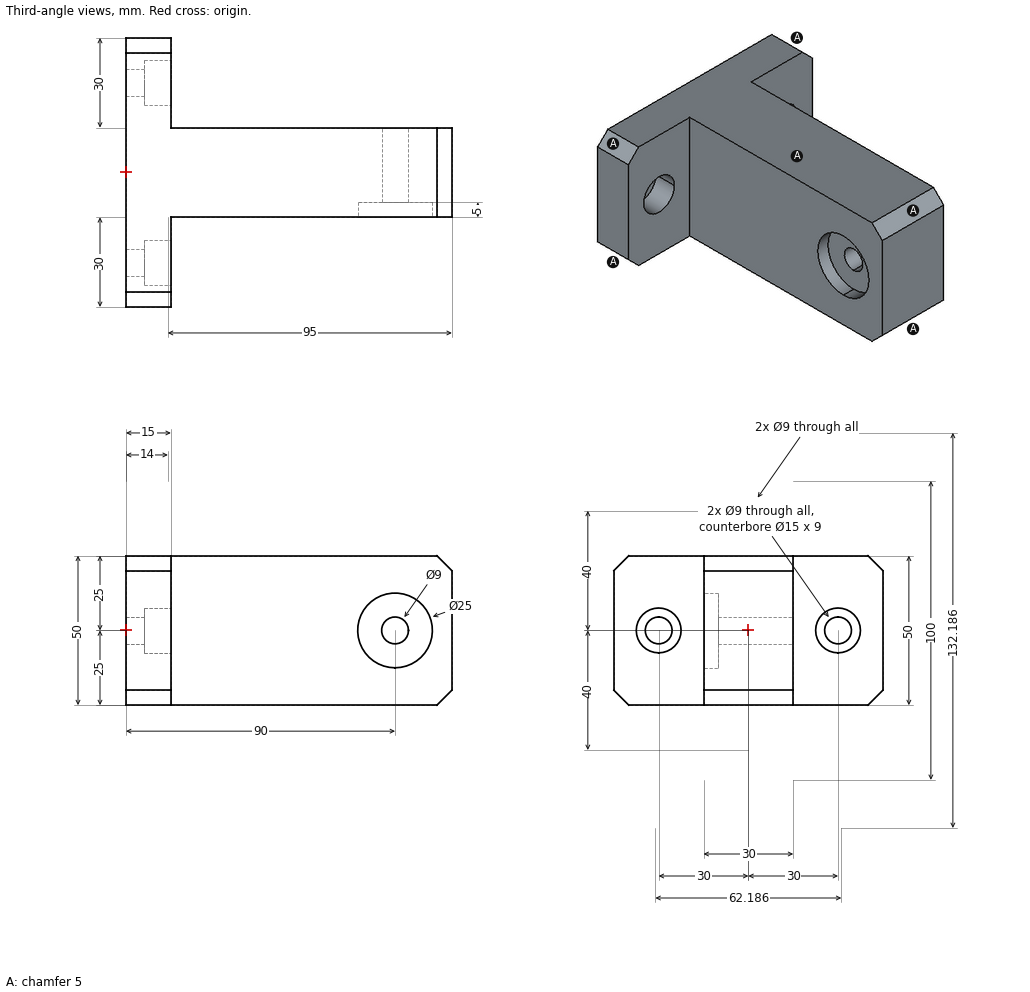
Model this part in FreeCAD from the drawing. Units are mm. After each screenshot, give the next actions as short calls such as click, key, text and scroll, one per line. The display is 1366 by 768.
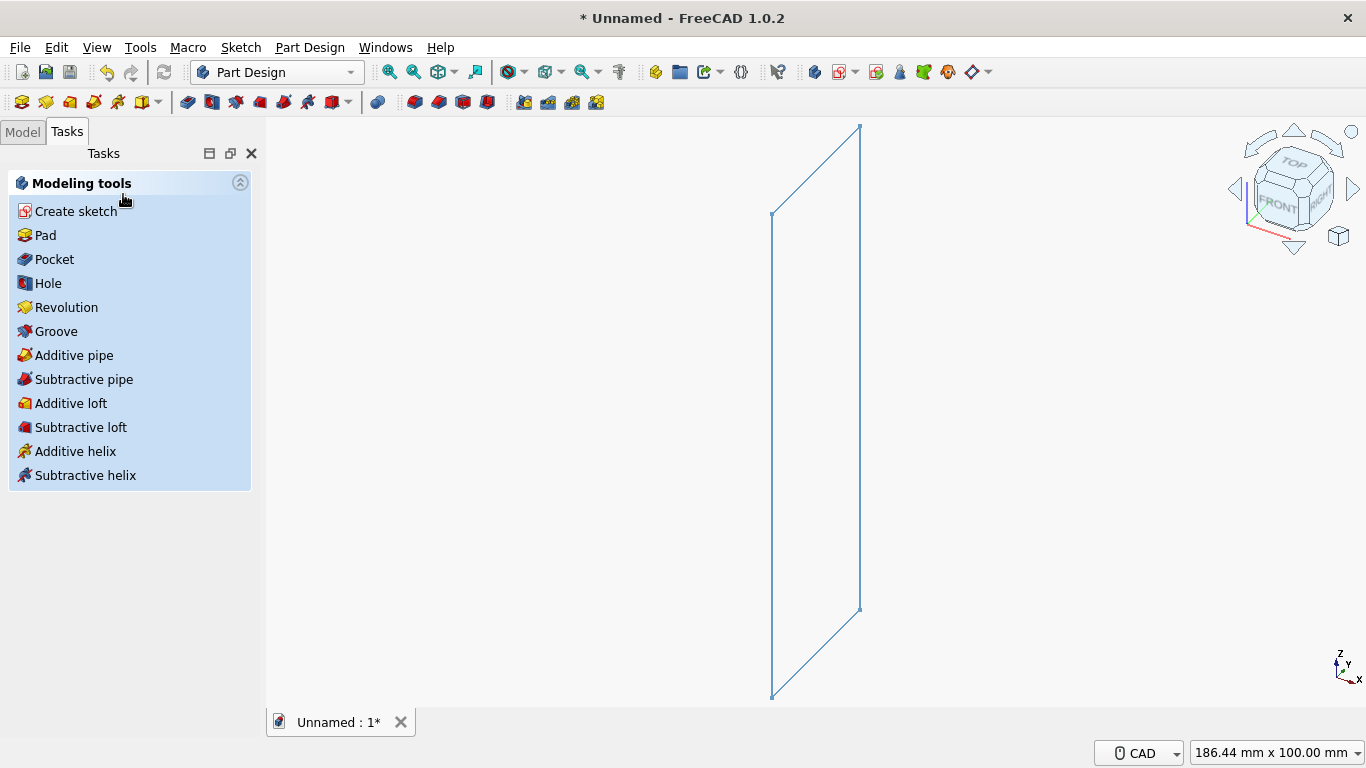
click(22, 102)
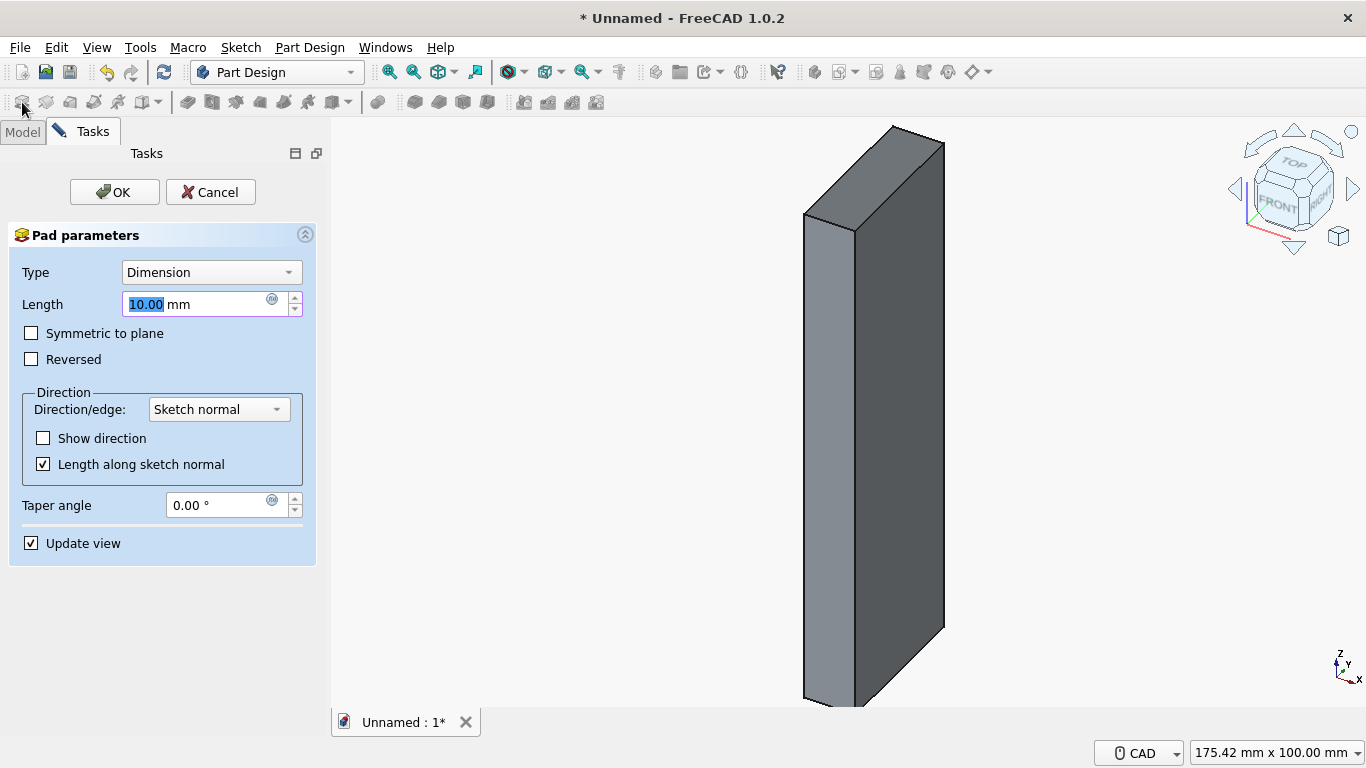
text(14)
key(Tab)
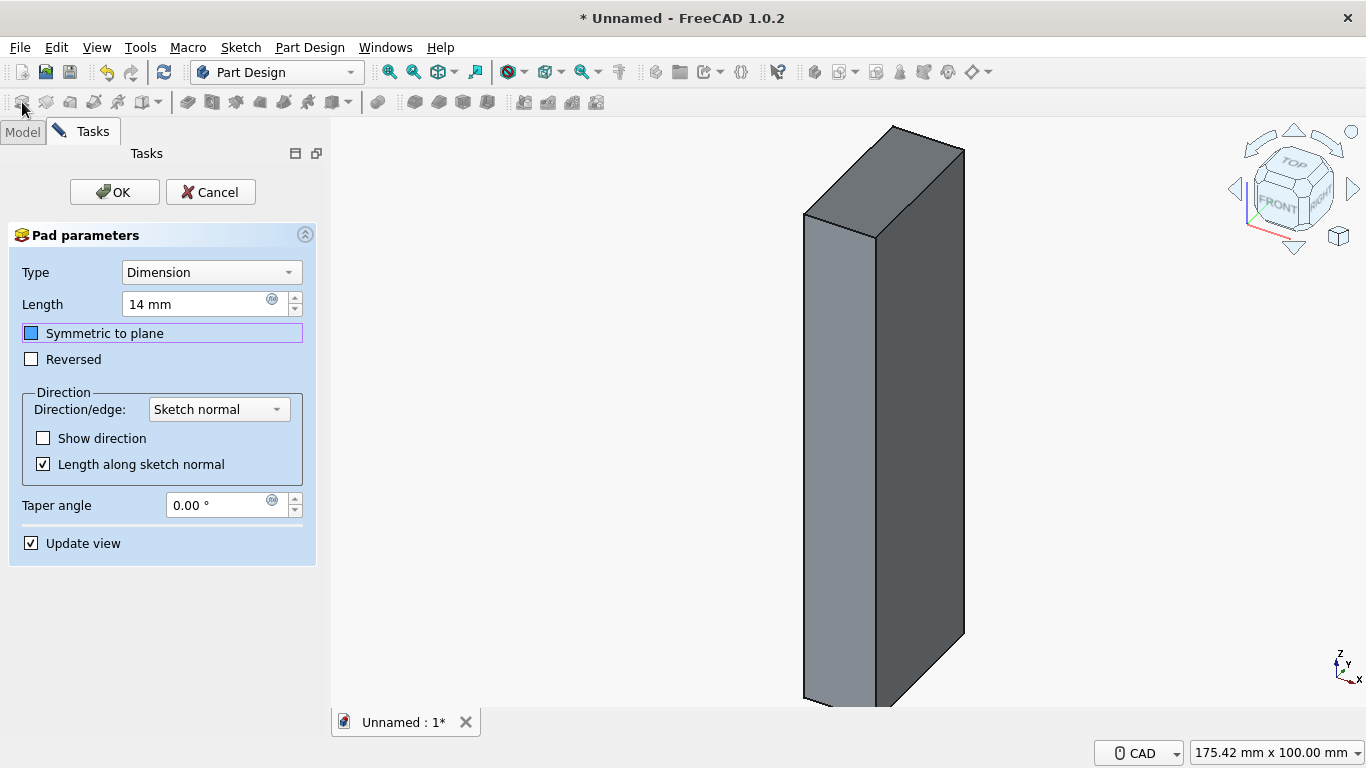
click(115, 192)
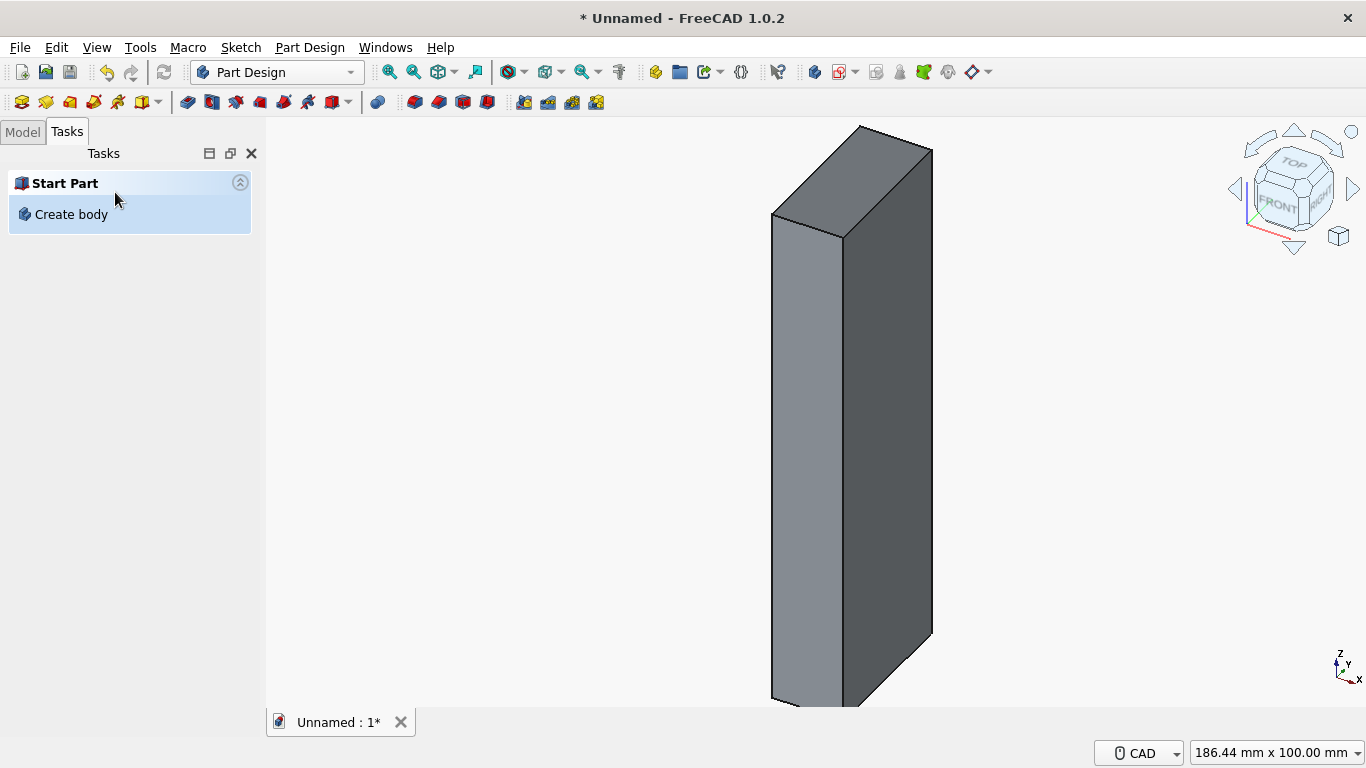
click(390, 72)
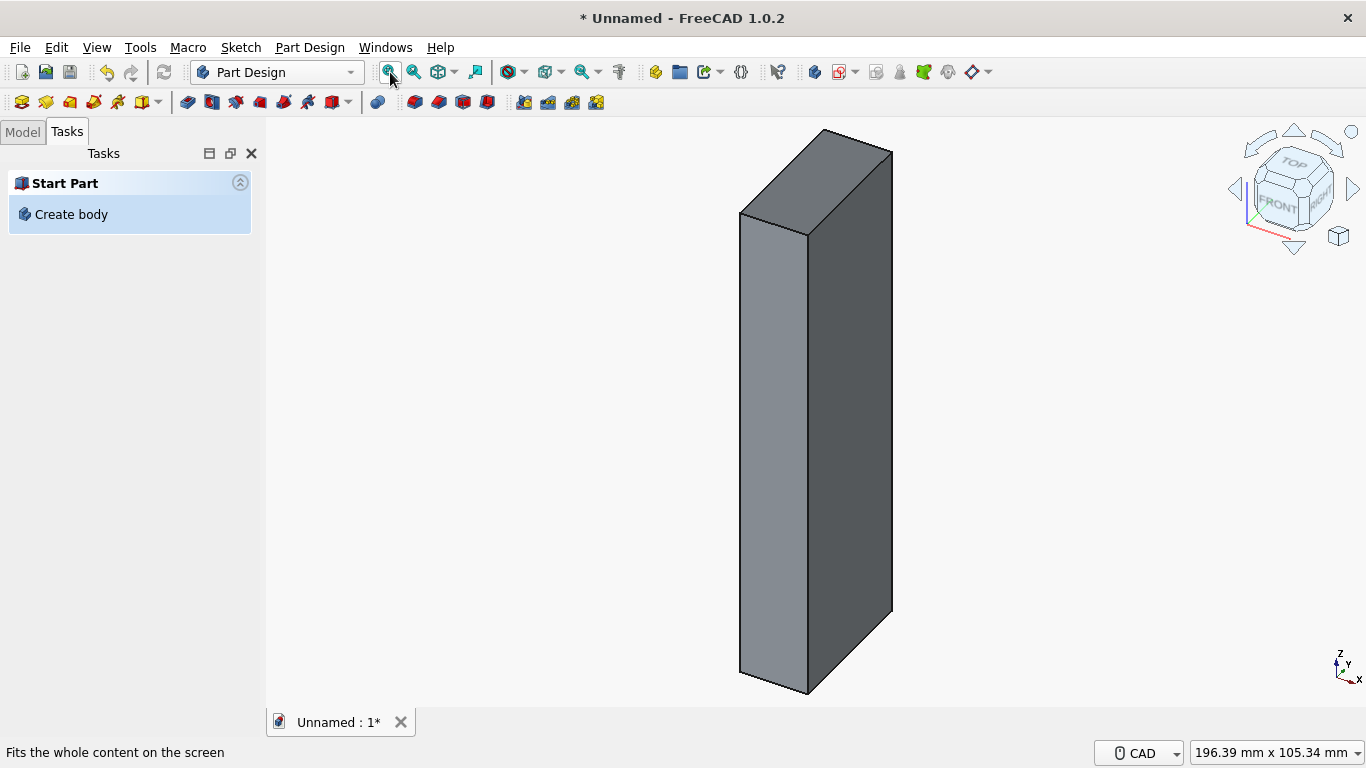
click(850, 553)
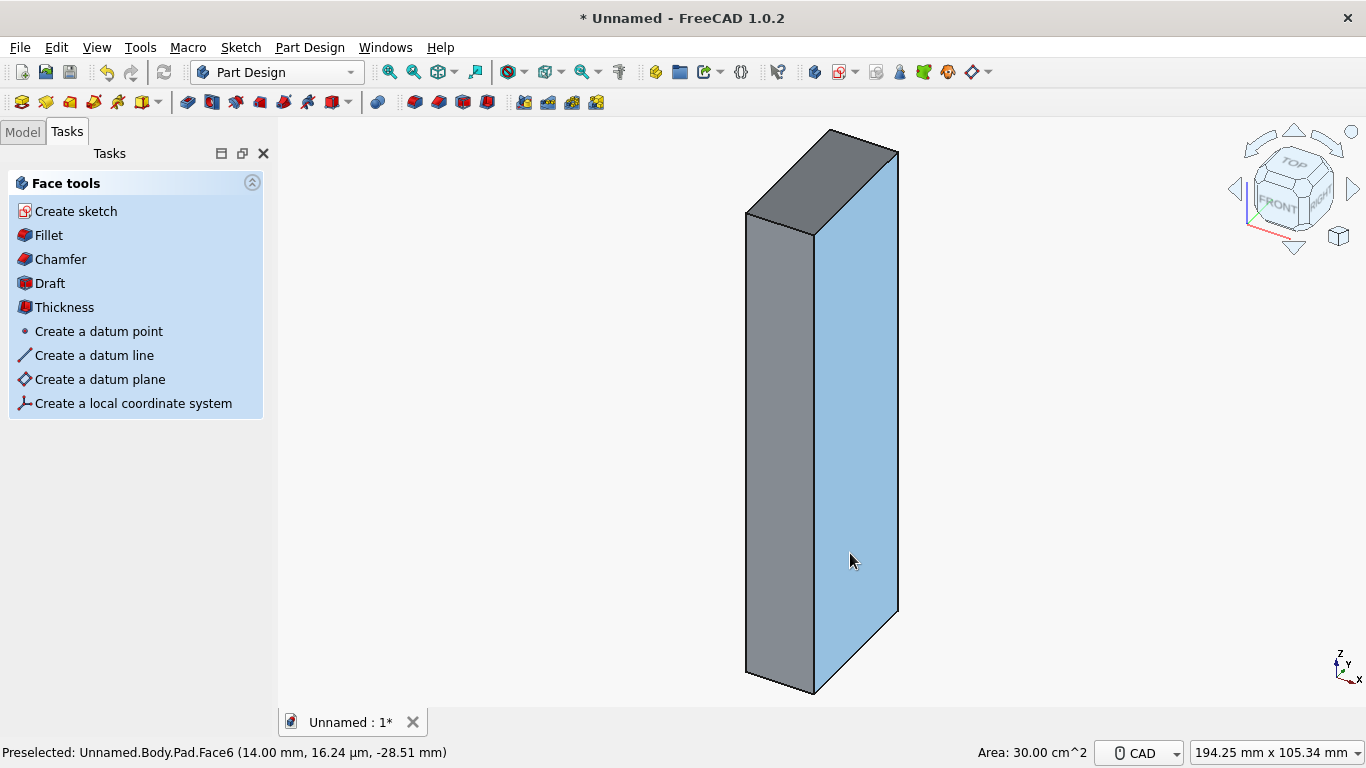
click(840, 72)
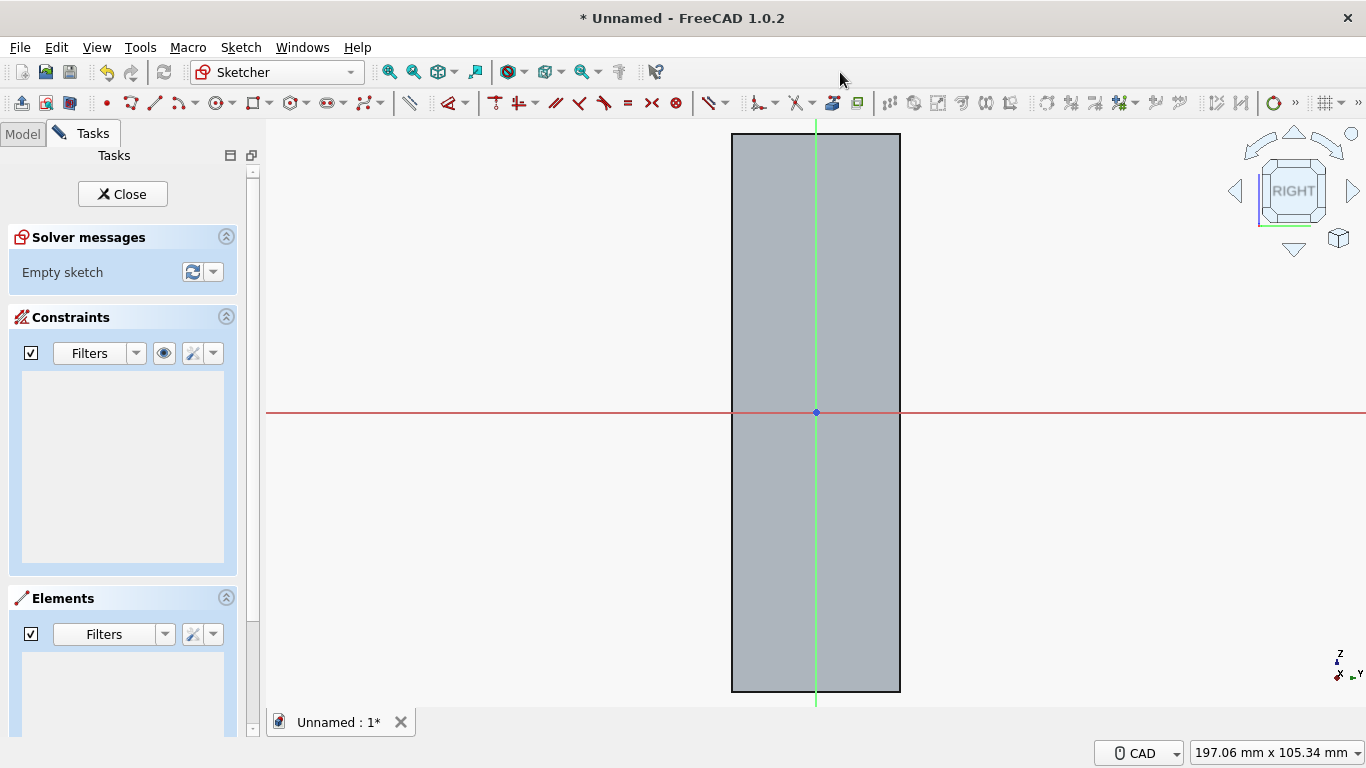
key(g)
key(v)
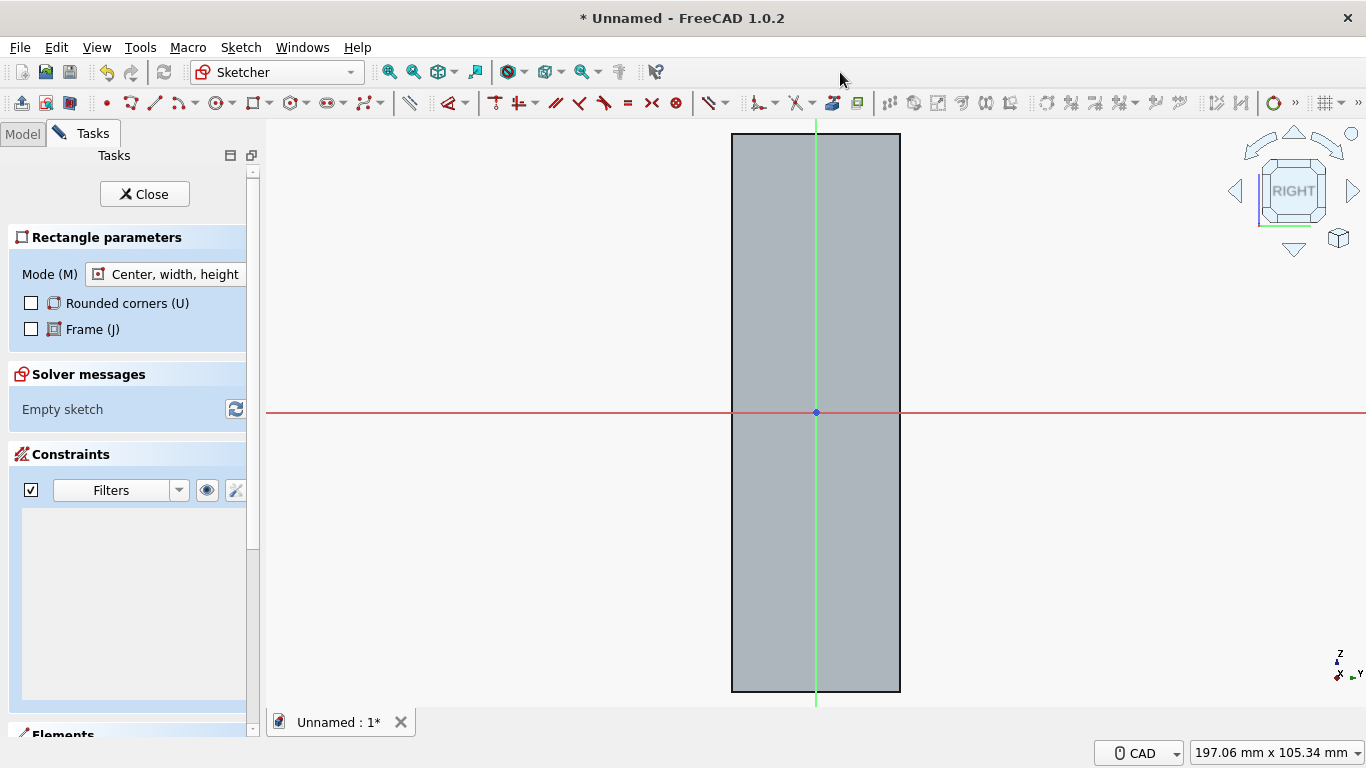
click(816, 413)
move(900, 273)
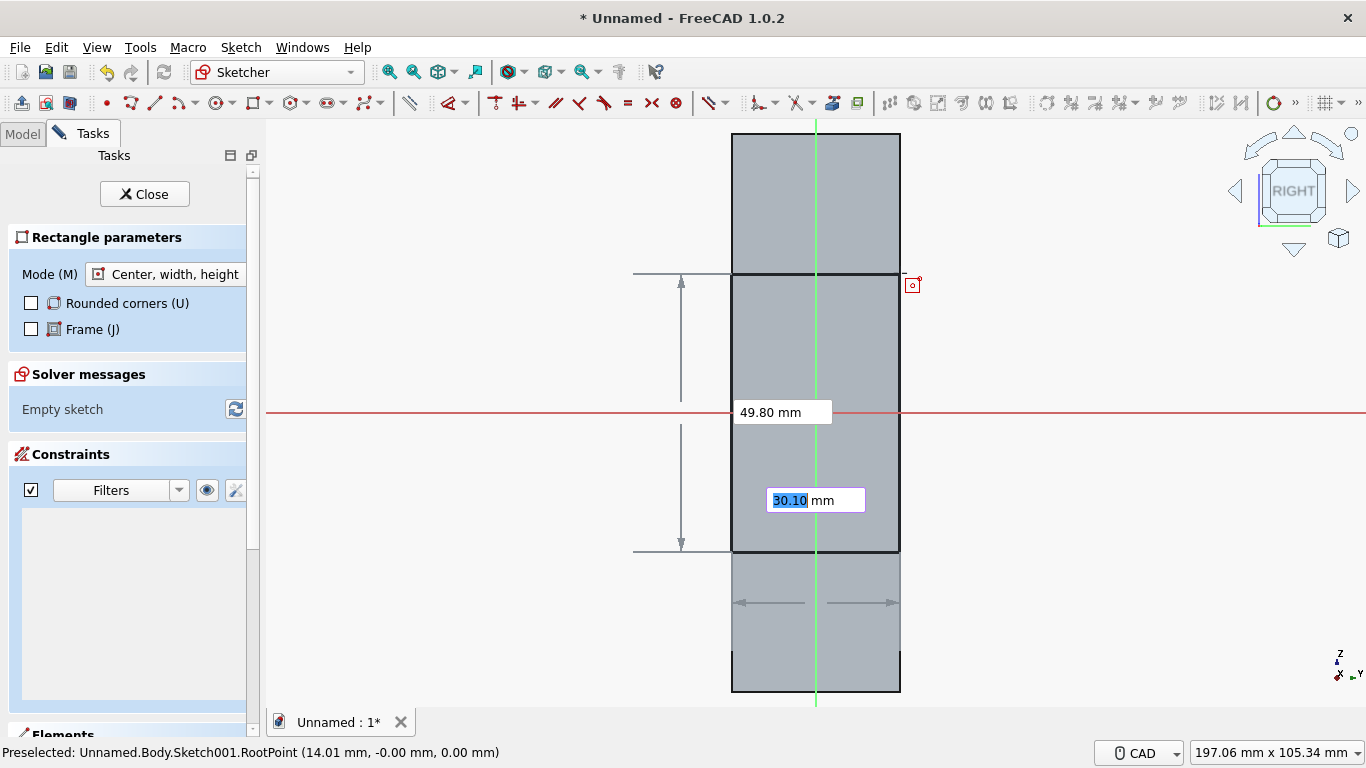
text(30)
key(Tab)
text(50)
key(Return)
key(Escape)